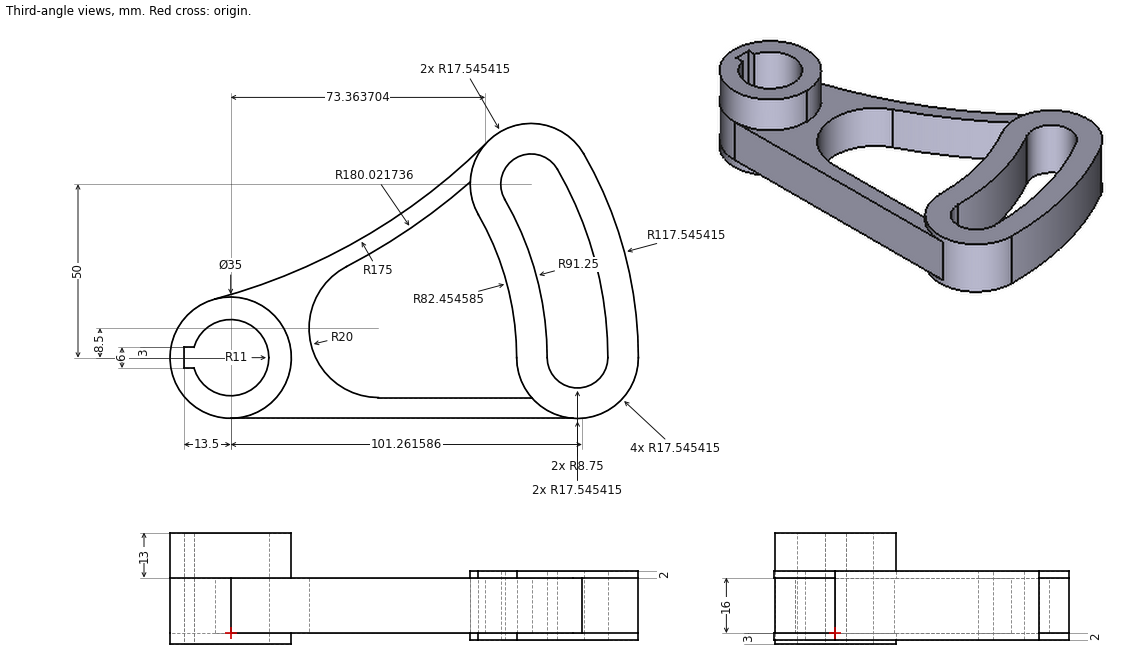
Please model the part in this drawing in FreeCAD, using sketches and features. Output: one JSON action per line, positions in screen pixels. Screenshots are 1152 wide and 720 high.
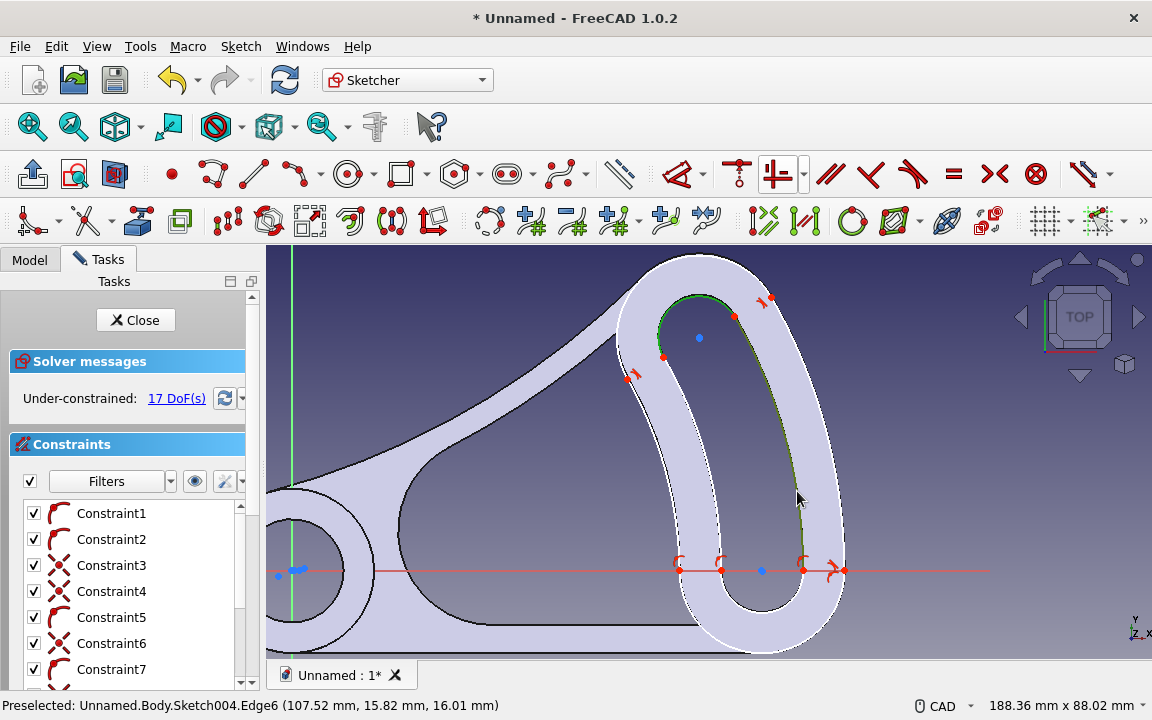
{"action": "left_click", "coordinate": [913, 174]}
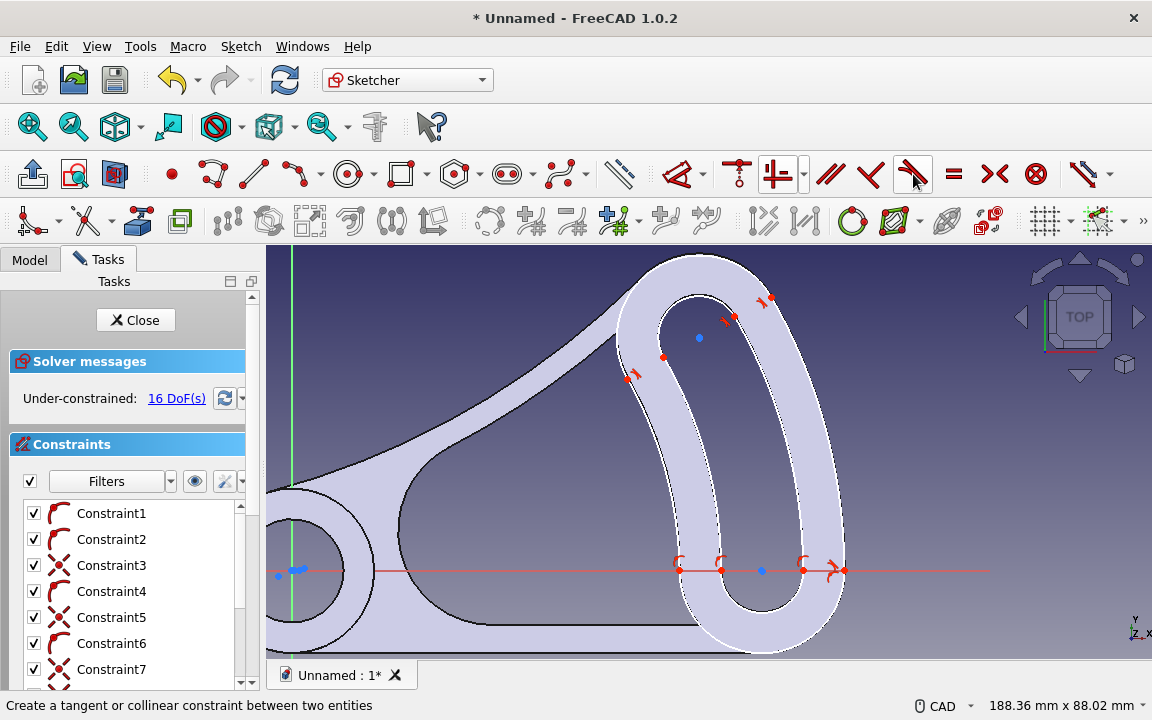
{"action": "left_click", "coordinate": [703, 296]}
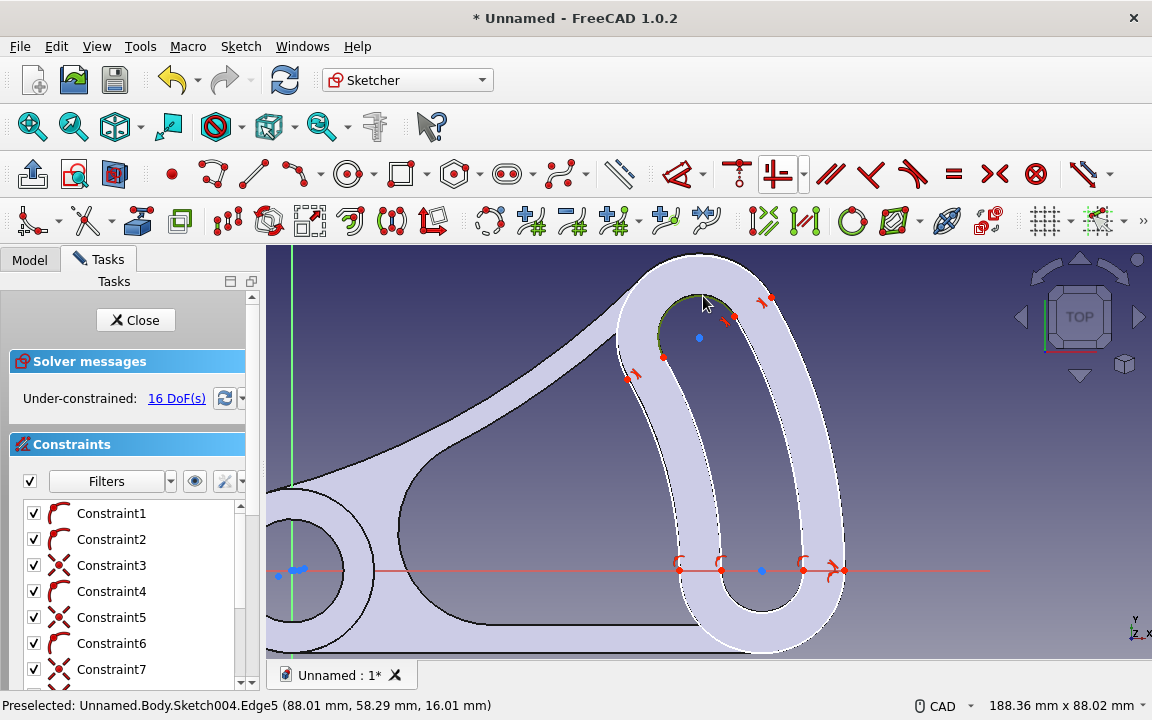
{"action": "left_click", "coordinate": [716, 504]}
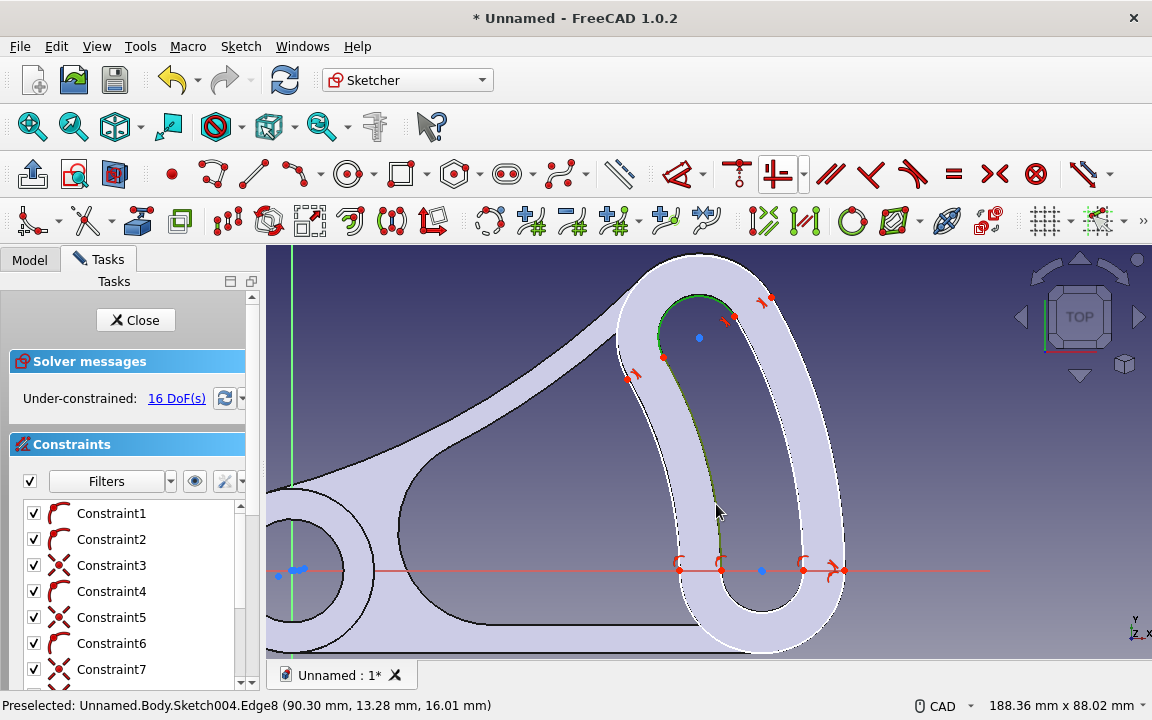
{"action": "left_click", "coordinate": [913, 174]}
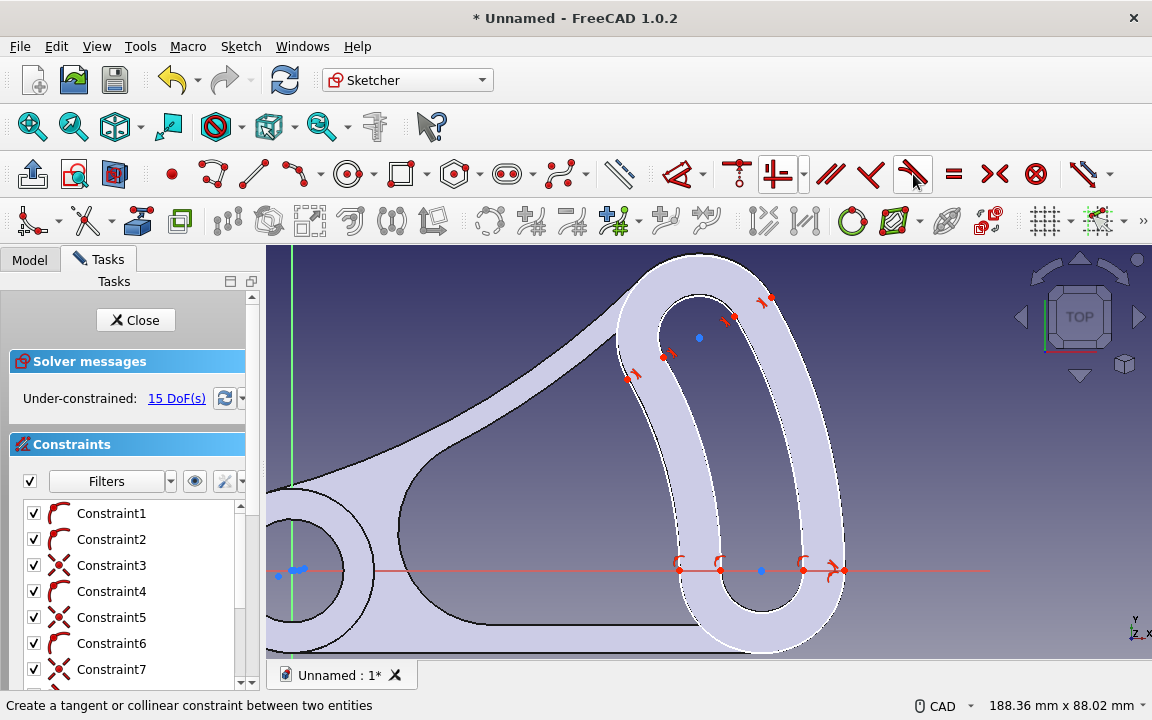
{"action": "left_click", "coordinate": [797, 491]}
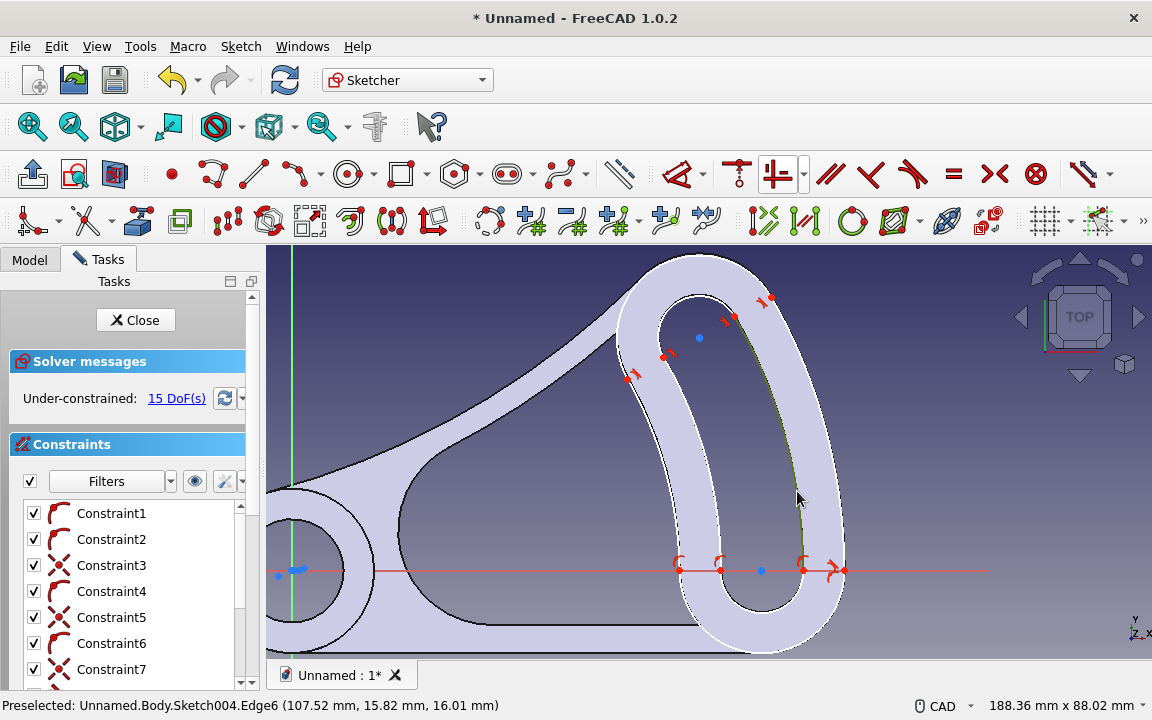
{"action": "left_click", "coordinate": [737, 605]}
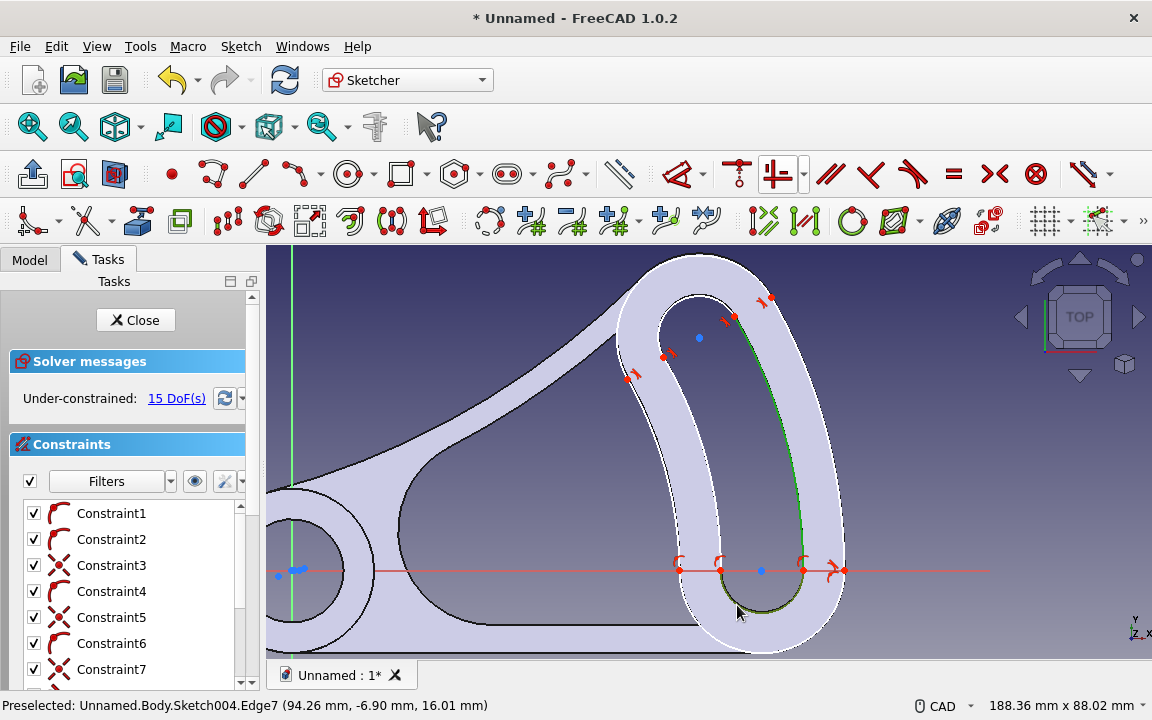
{"action": "left_click", "coordinate": [913, 174]}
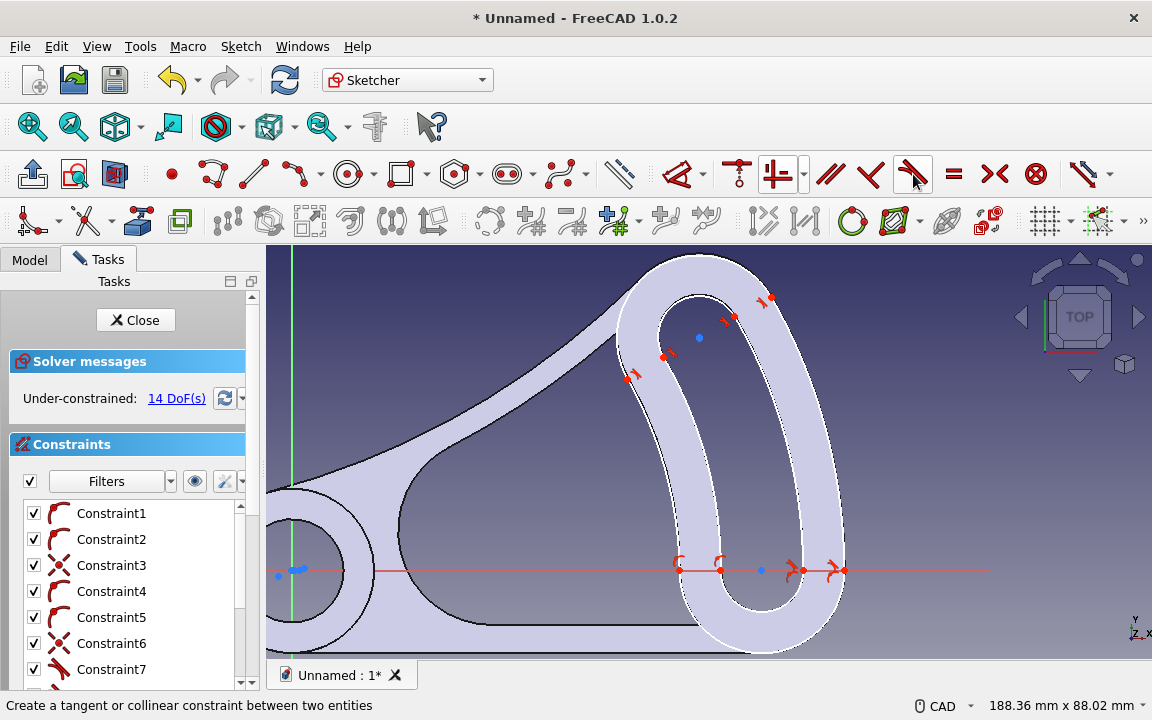
{"action": "left_click", "coordinate": [838, 485]}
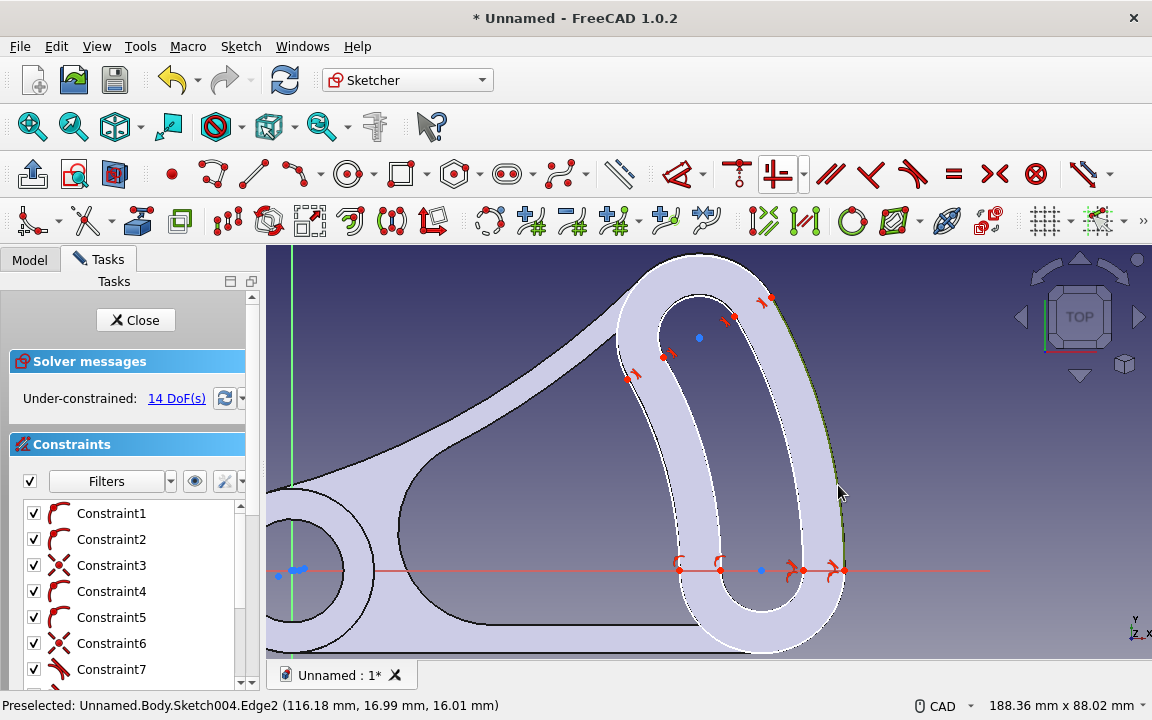
{"action": "left_click", "coordinate": [674, 511]}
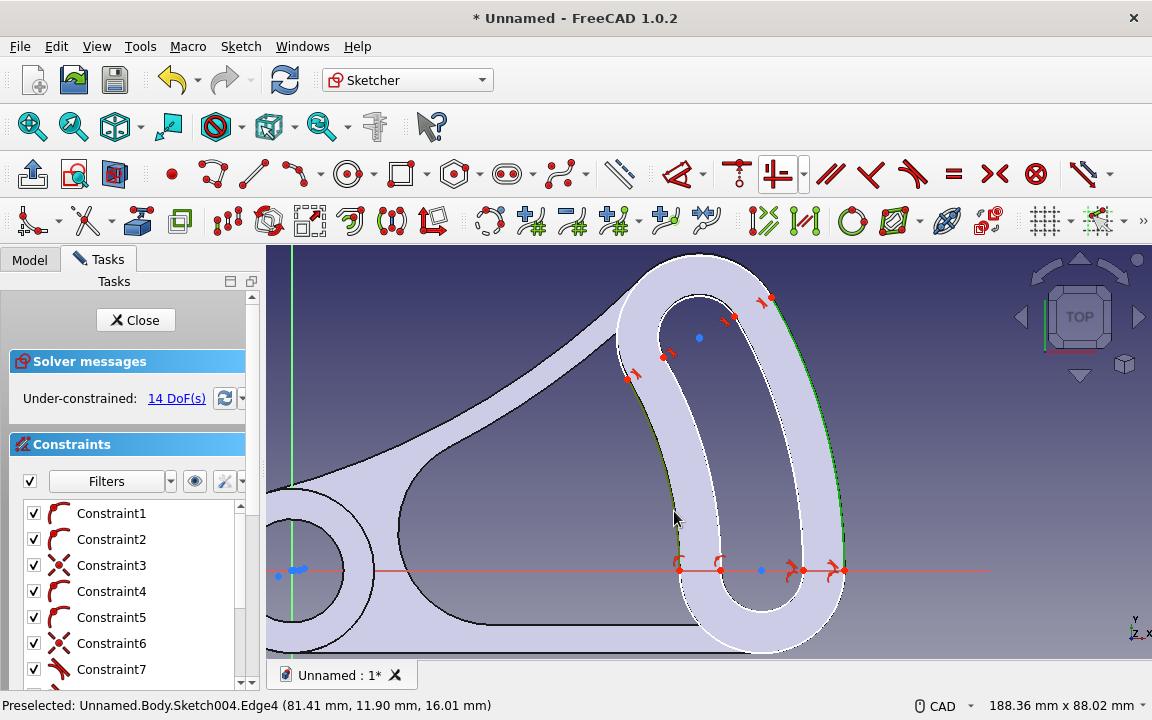
{"action": "left_click", "coordinate": [737, 174]}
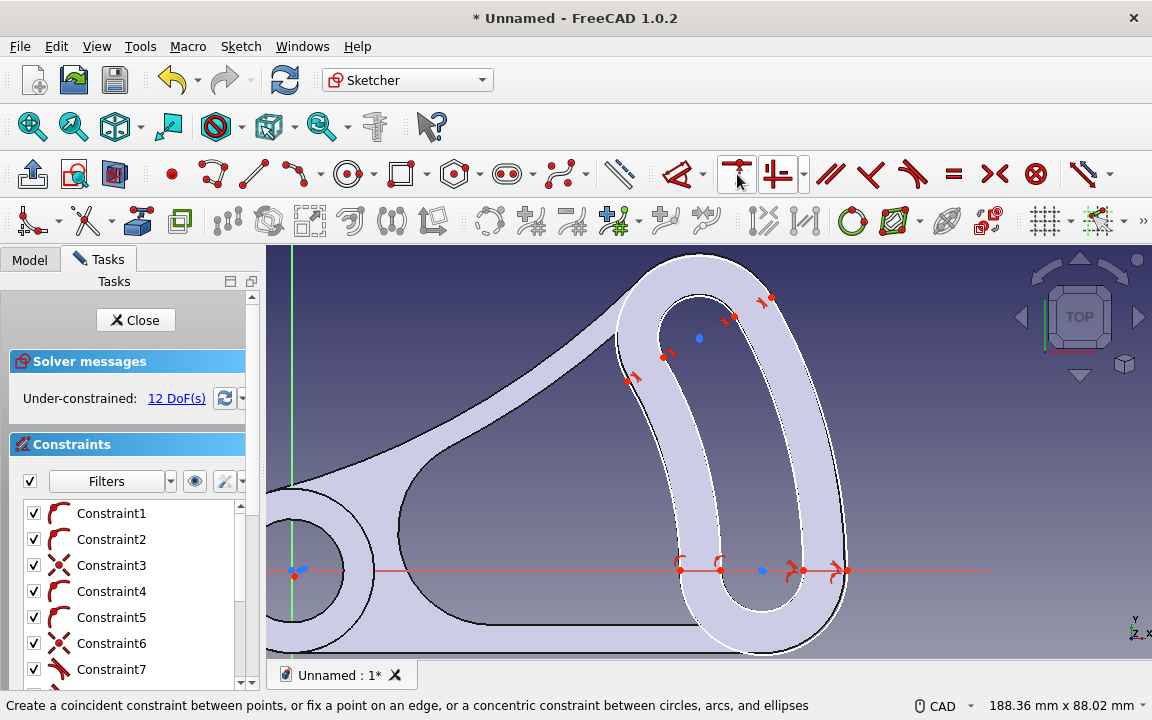
{"action": "left_click", "coordinate": [623, 306]}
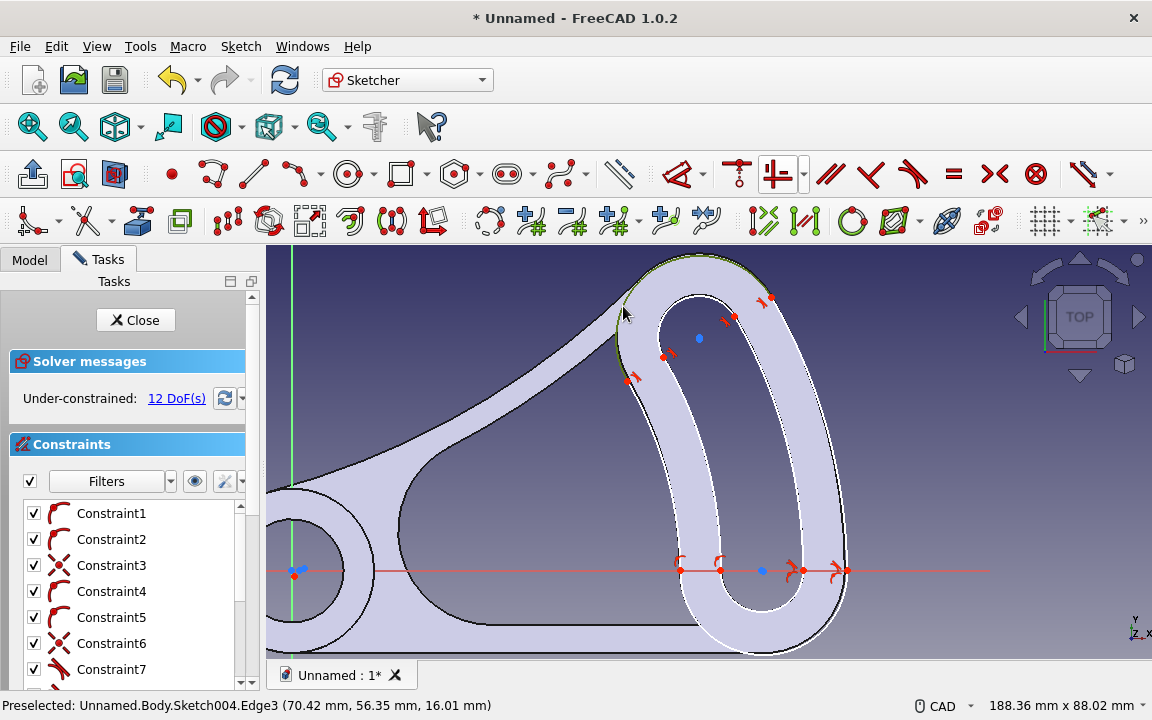
{"action": "left_click", "coordinate": [703, 296]}